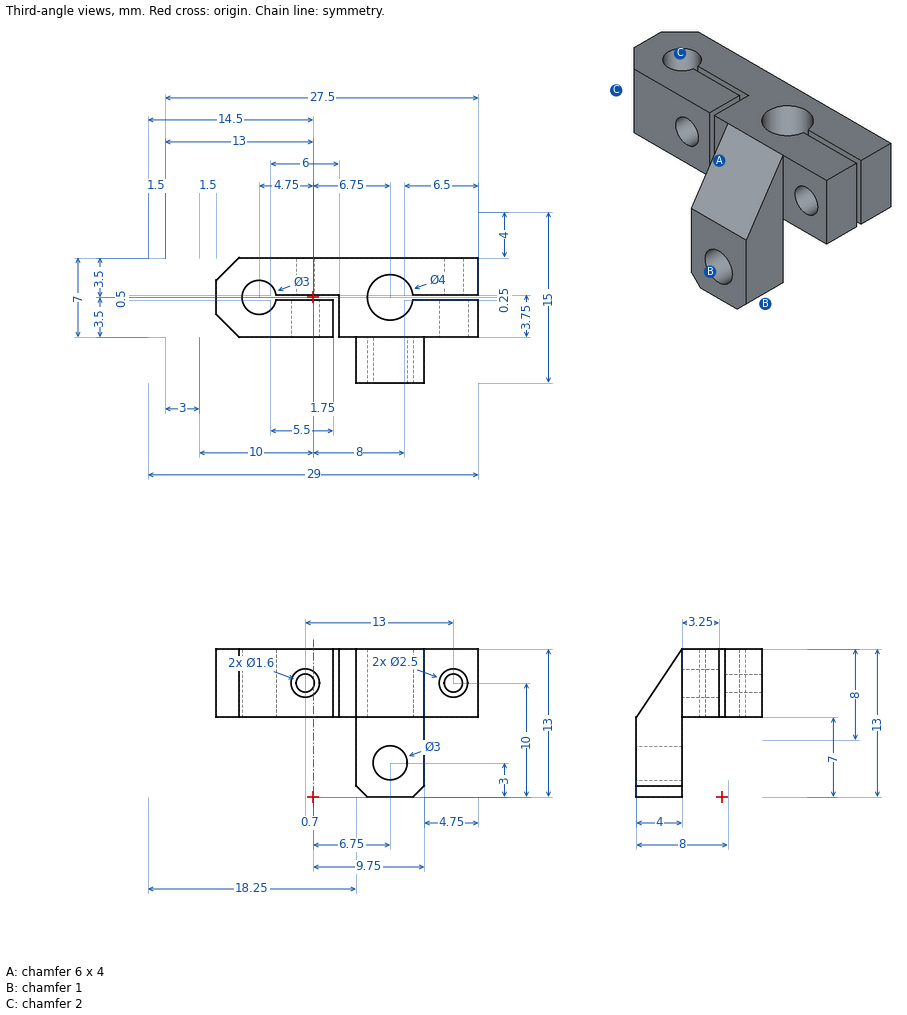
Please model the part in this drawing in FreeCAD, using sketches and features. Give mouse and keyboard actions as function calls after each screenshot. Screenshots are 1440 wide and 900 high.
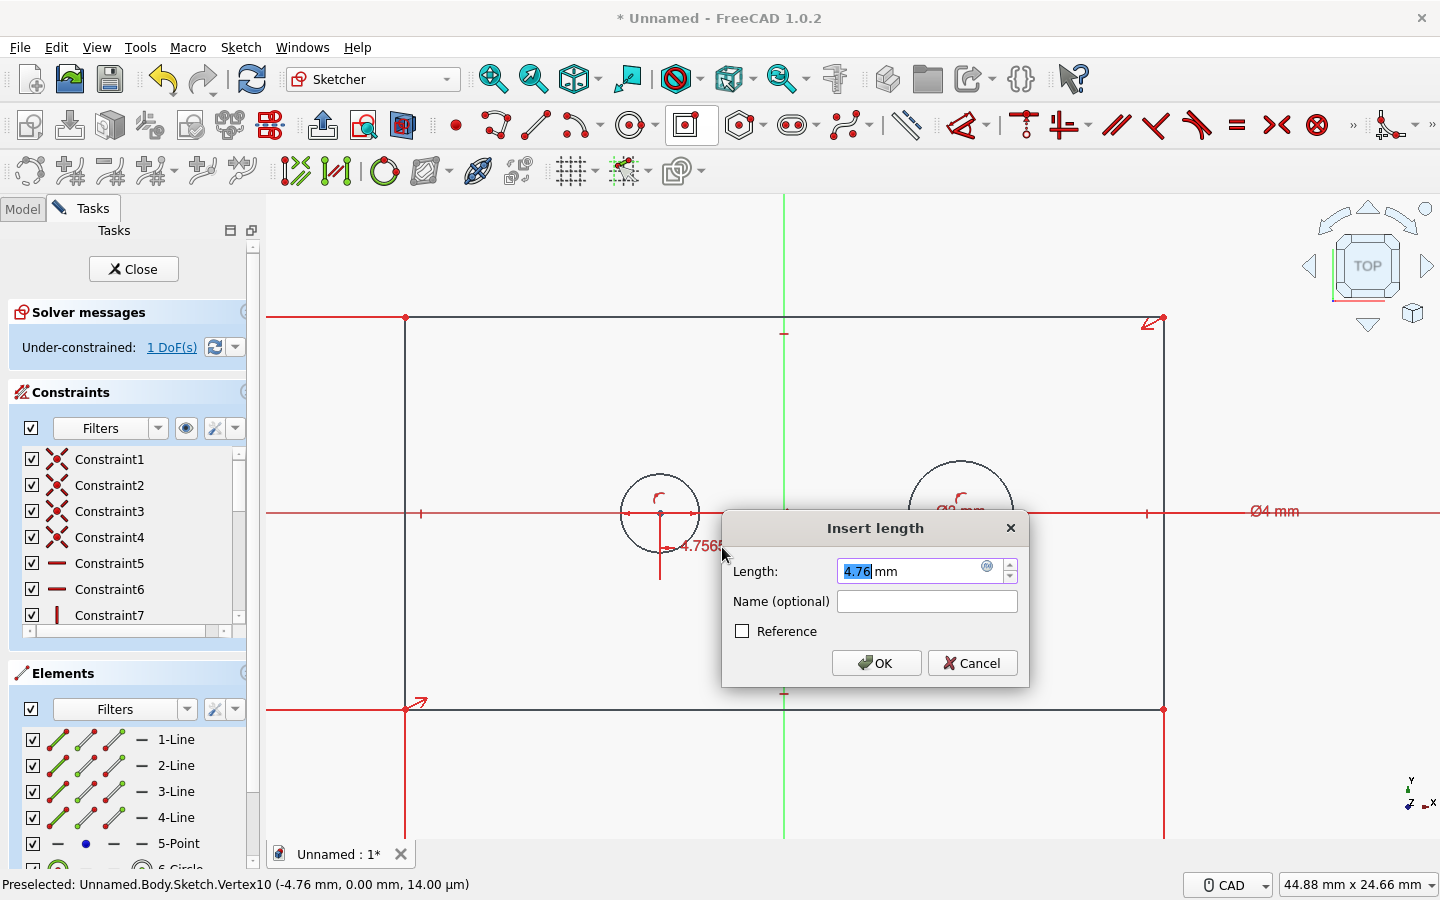
text(4.75)
key(Return)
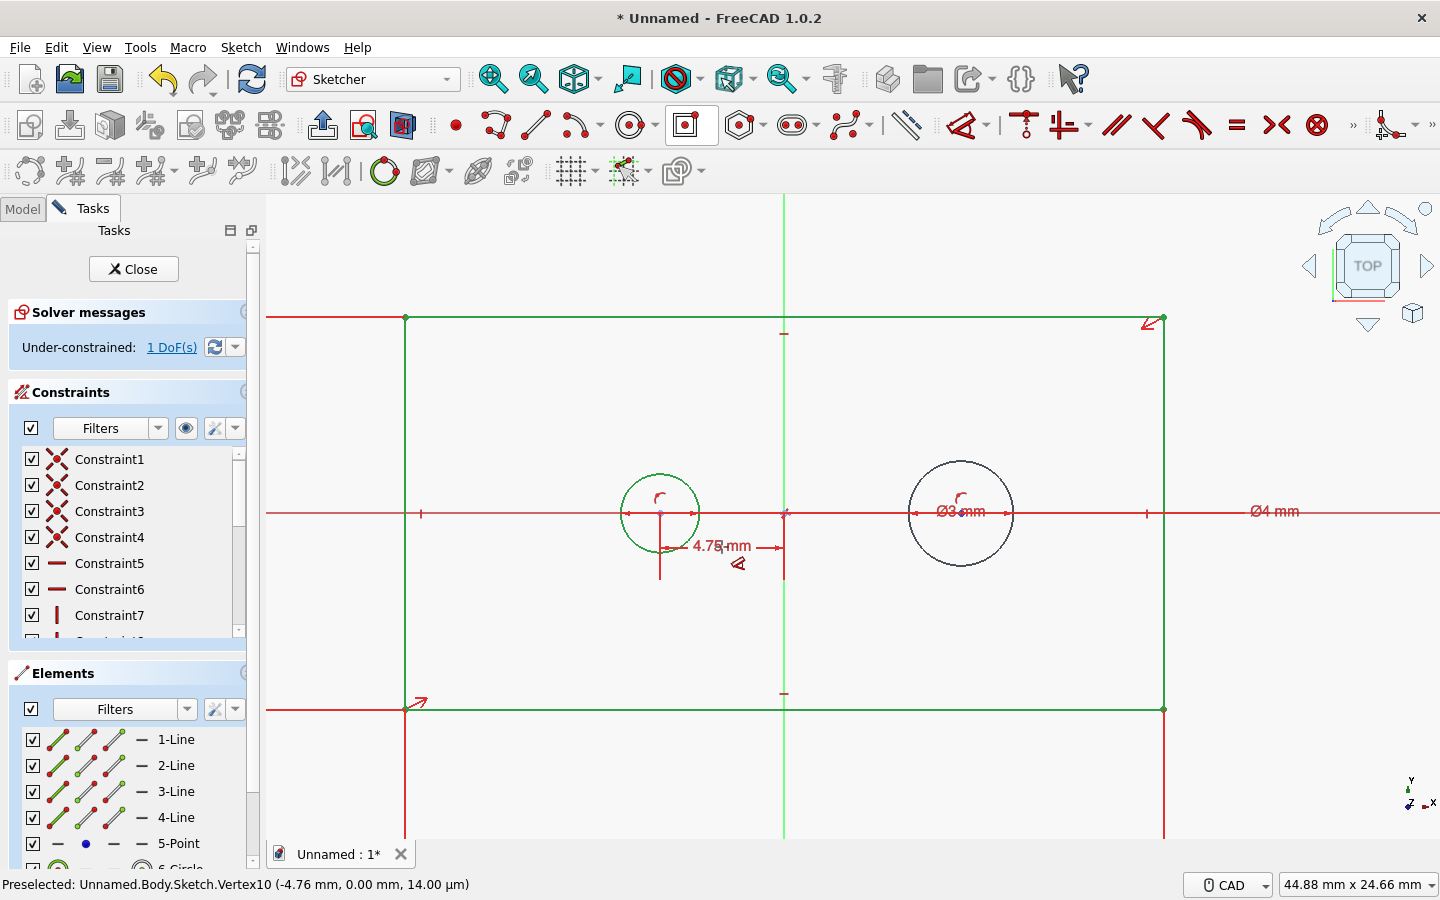
click(961, 513)
click(873, 547)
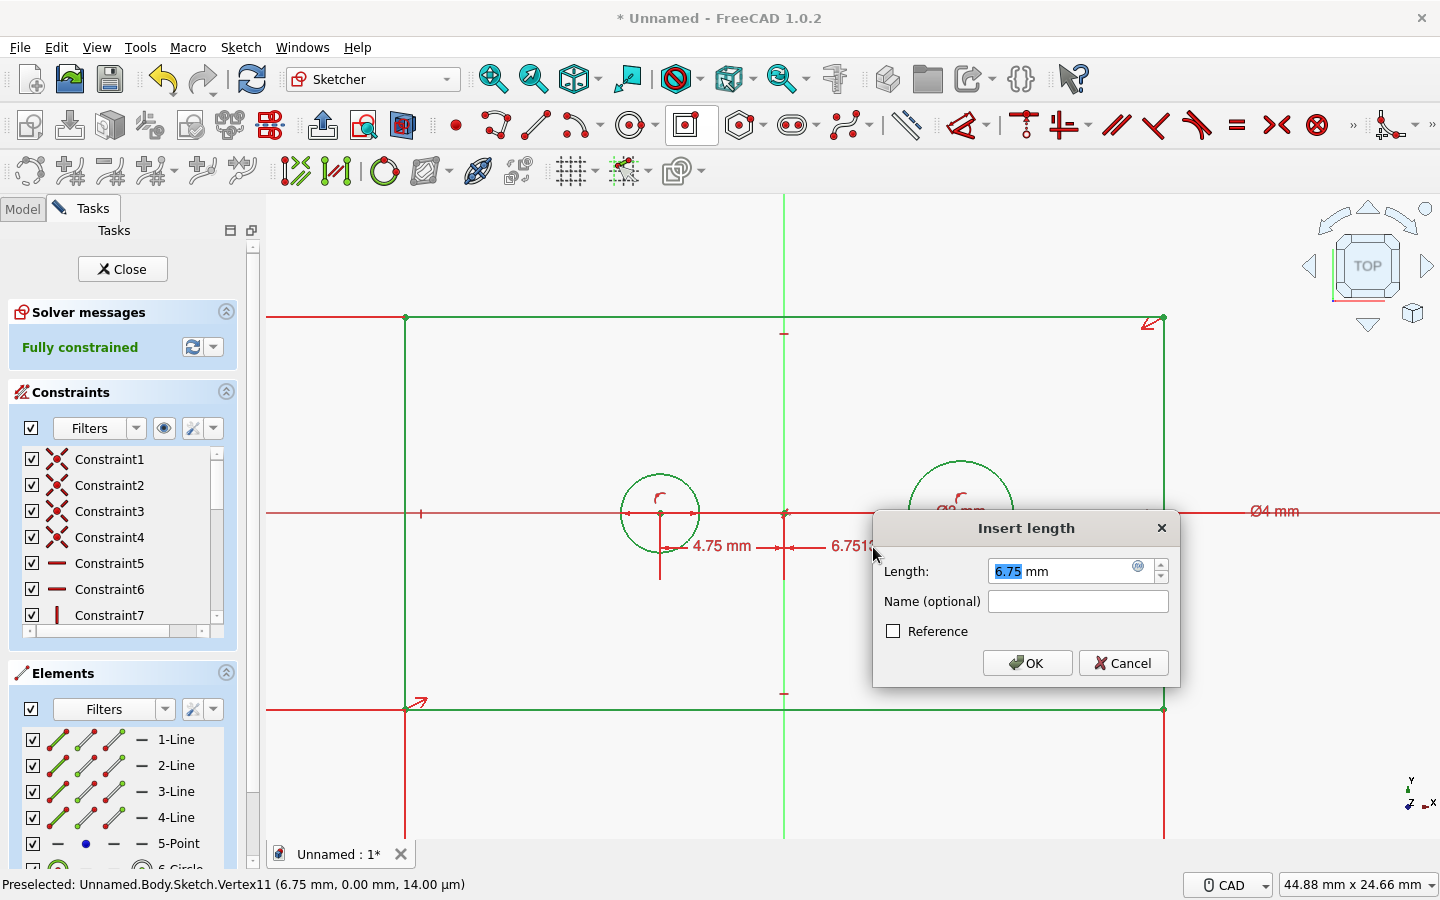
text(6.75)
key(Return)
key(Escape)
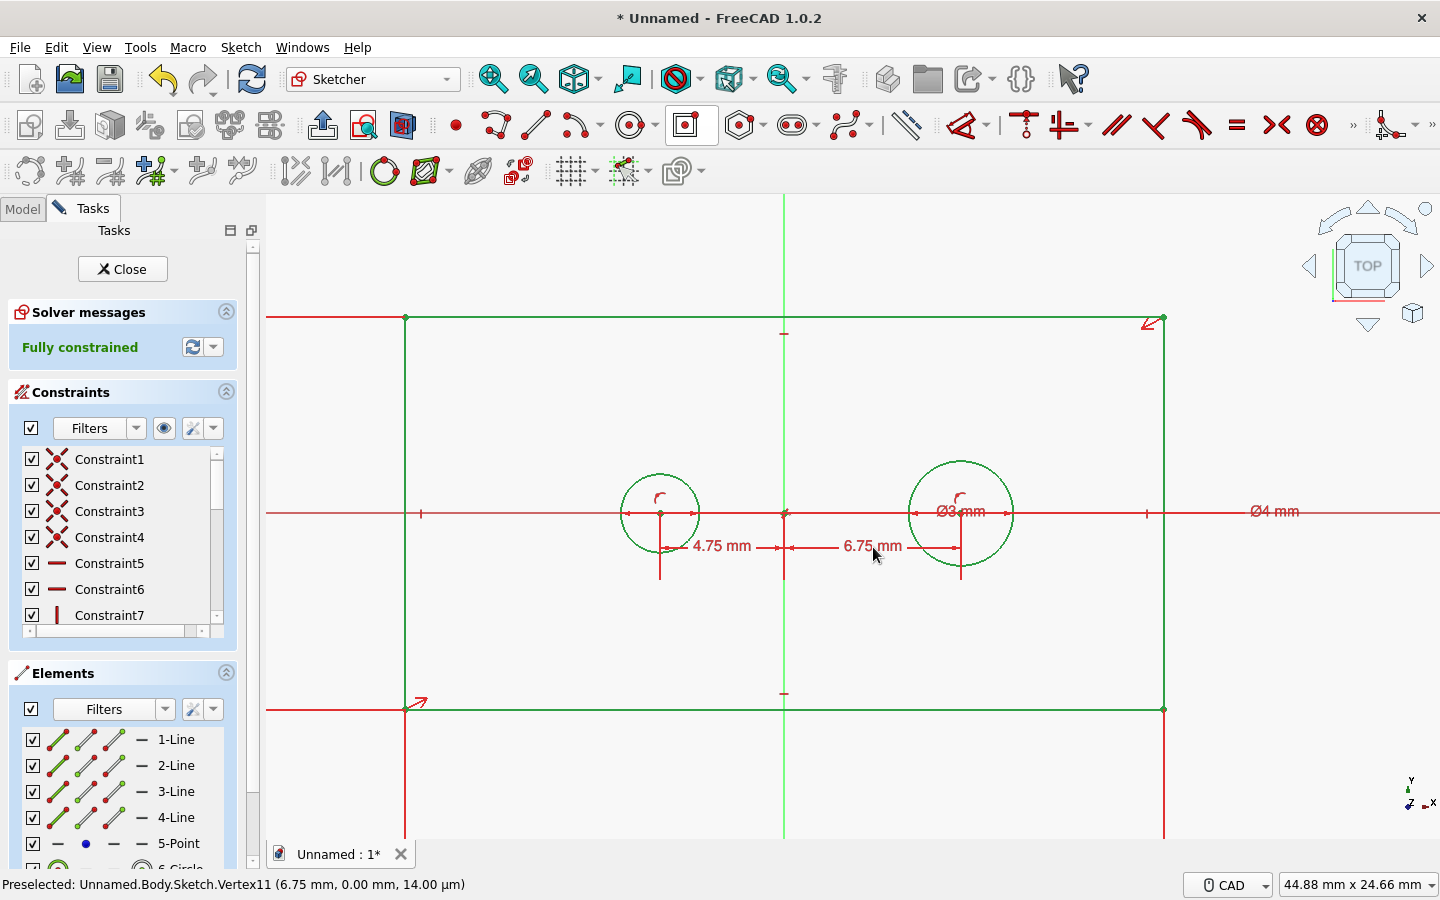
click(123, 269)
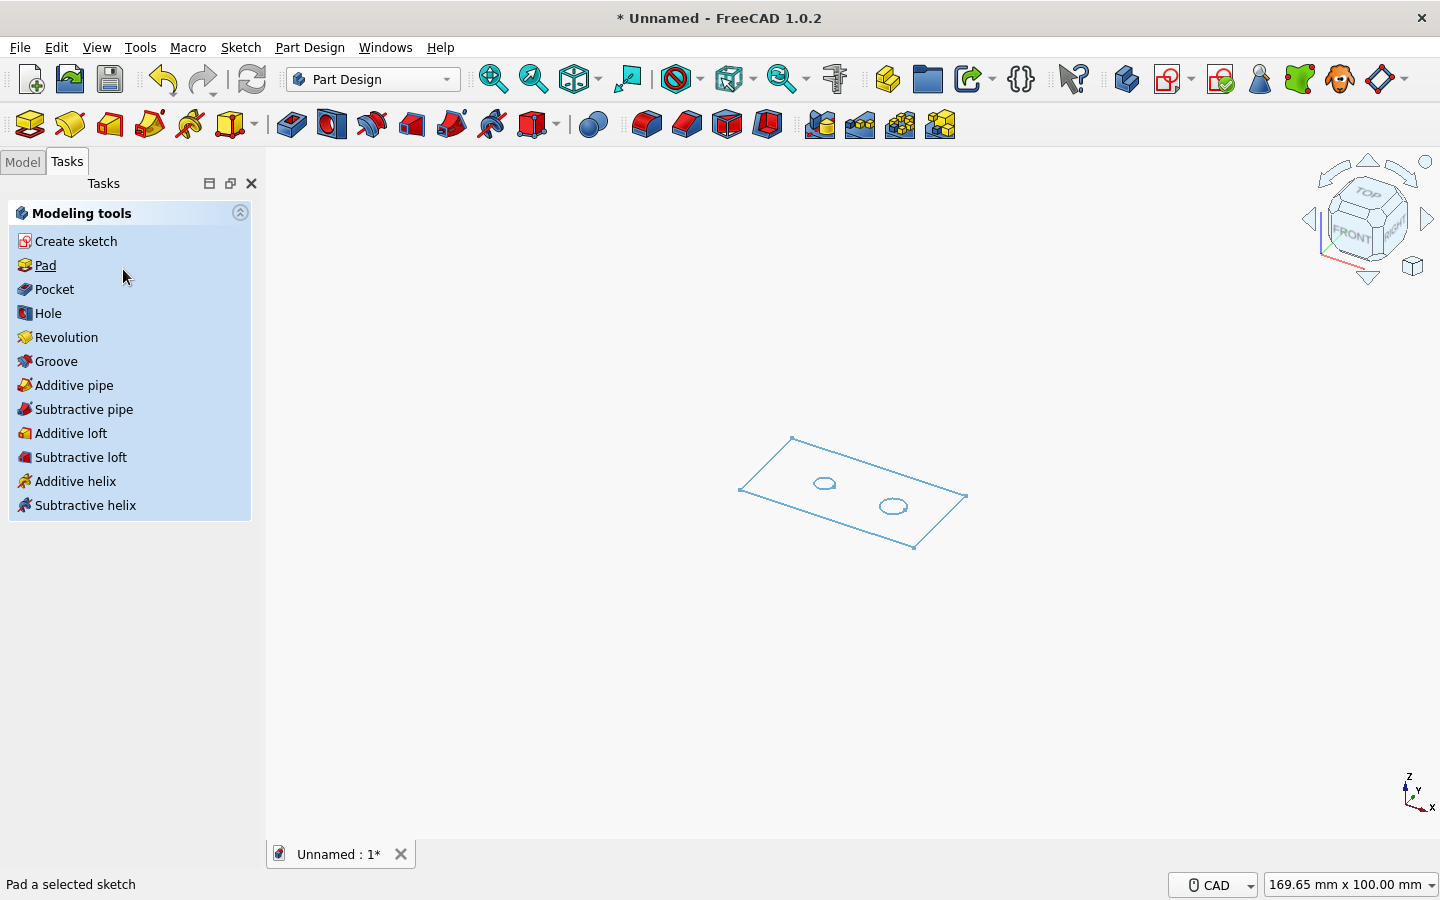
click(30, 124)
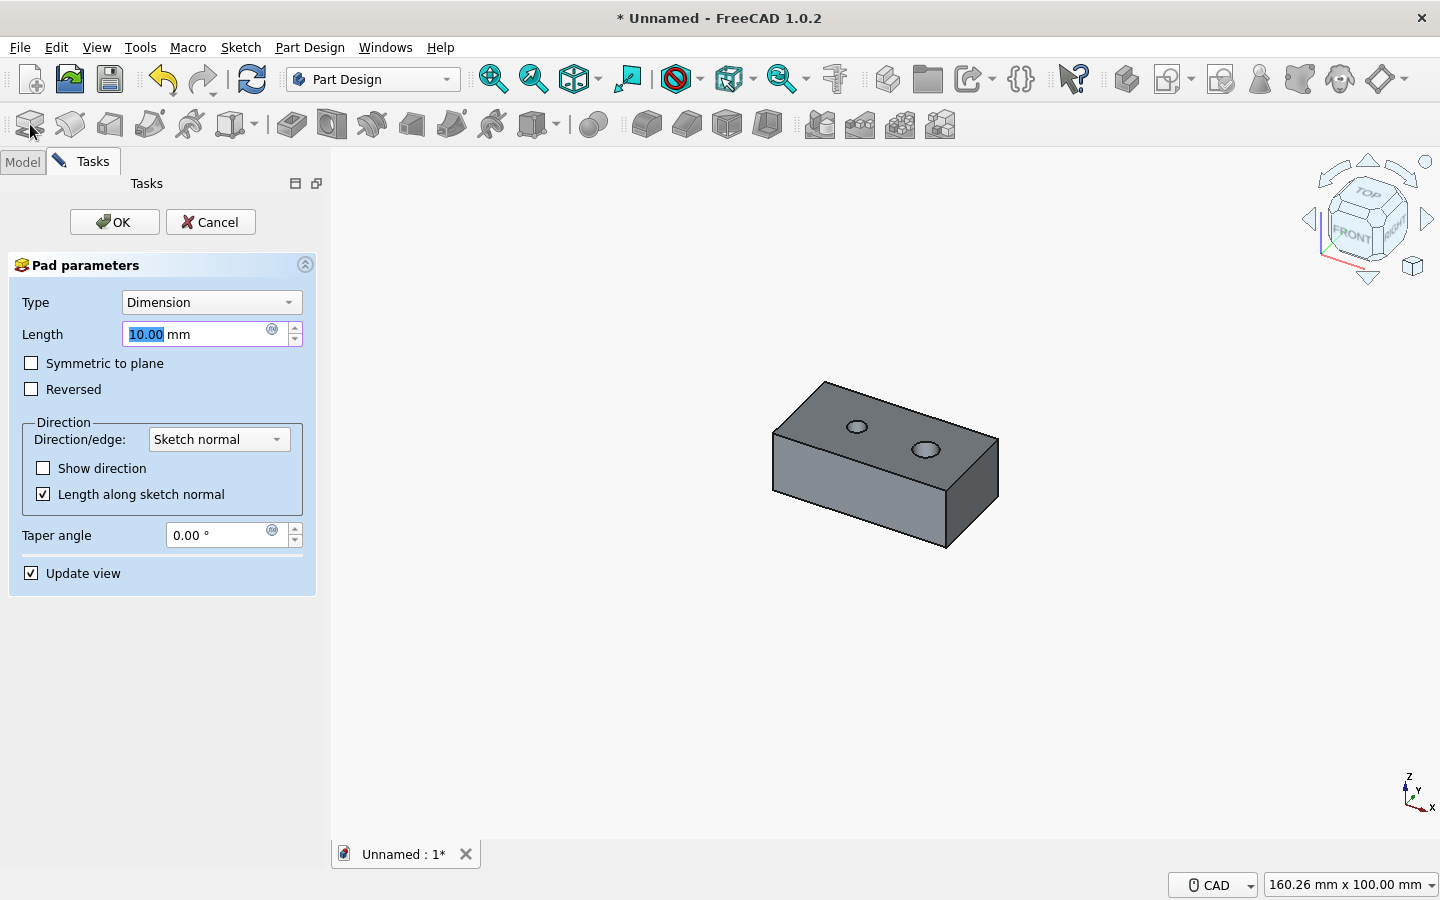
text(13)
key(Tab)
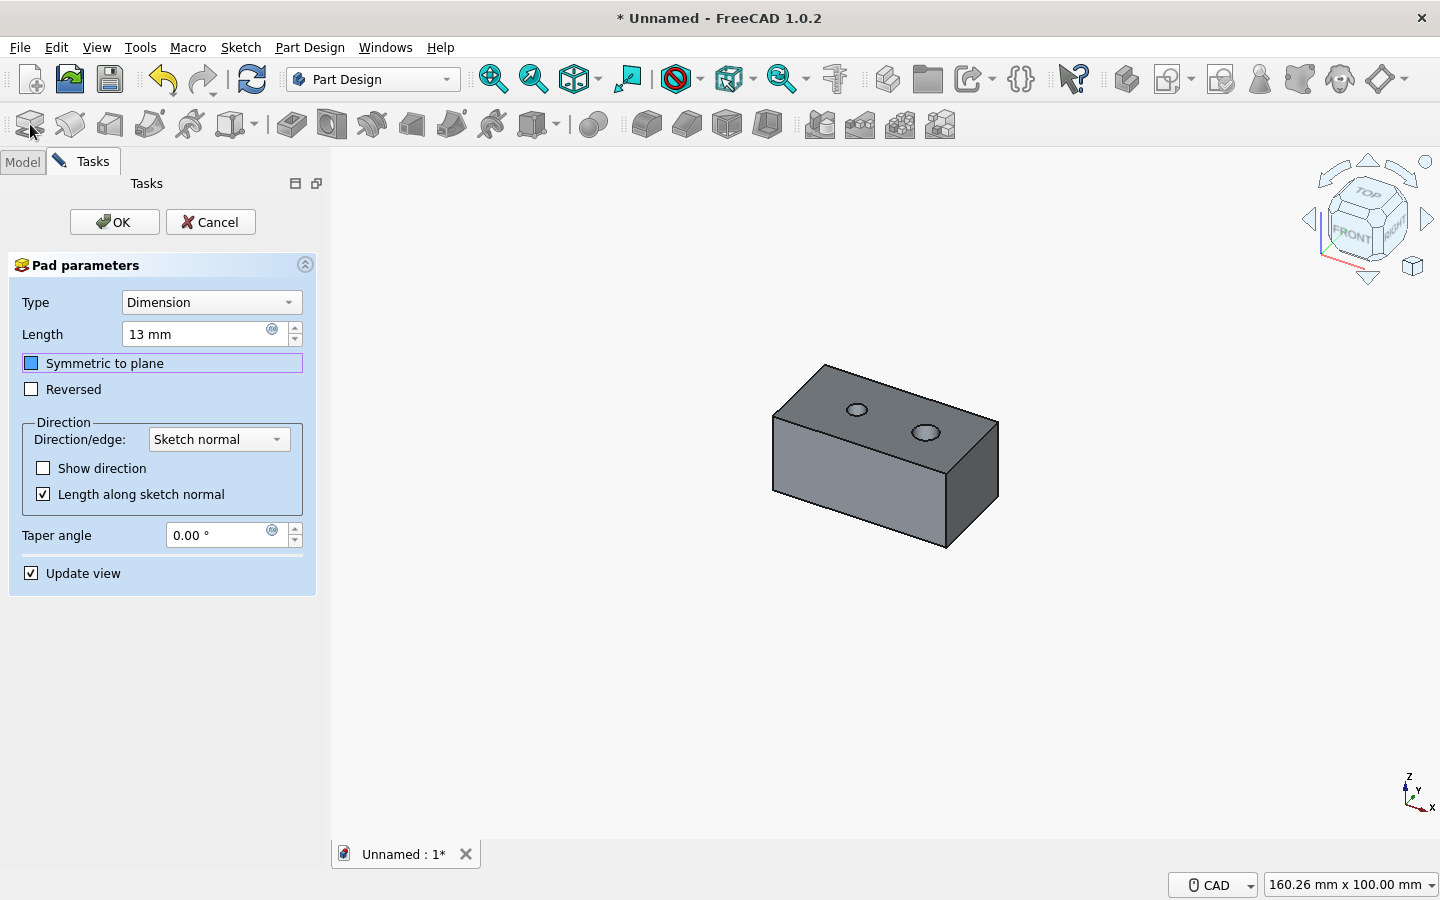
click(115, 222)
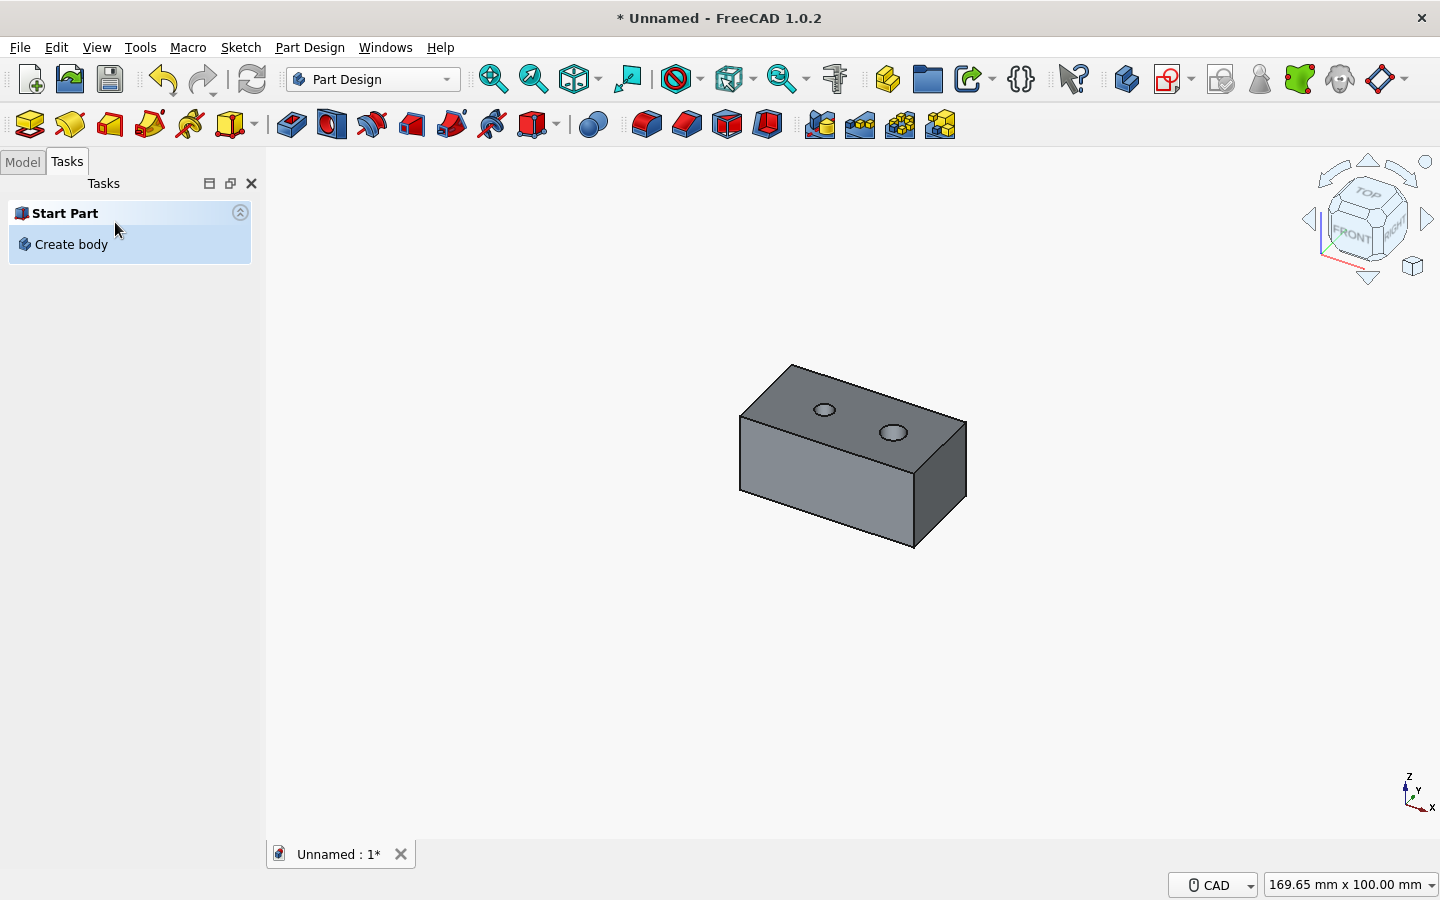
click(494, 80)